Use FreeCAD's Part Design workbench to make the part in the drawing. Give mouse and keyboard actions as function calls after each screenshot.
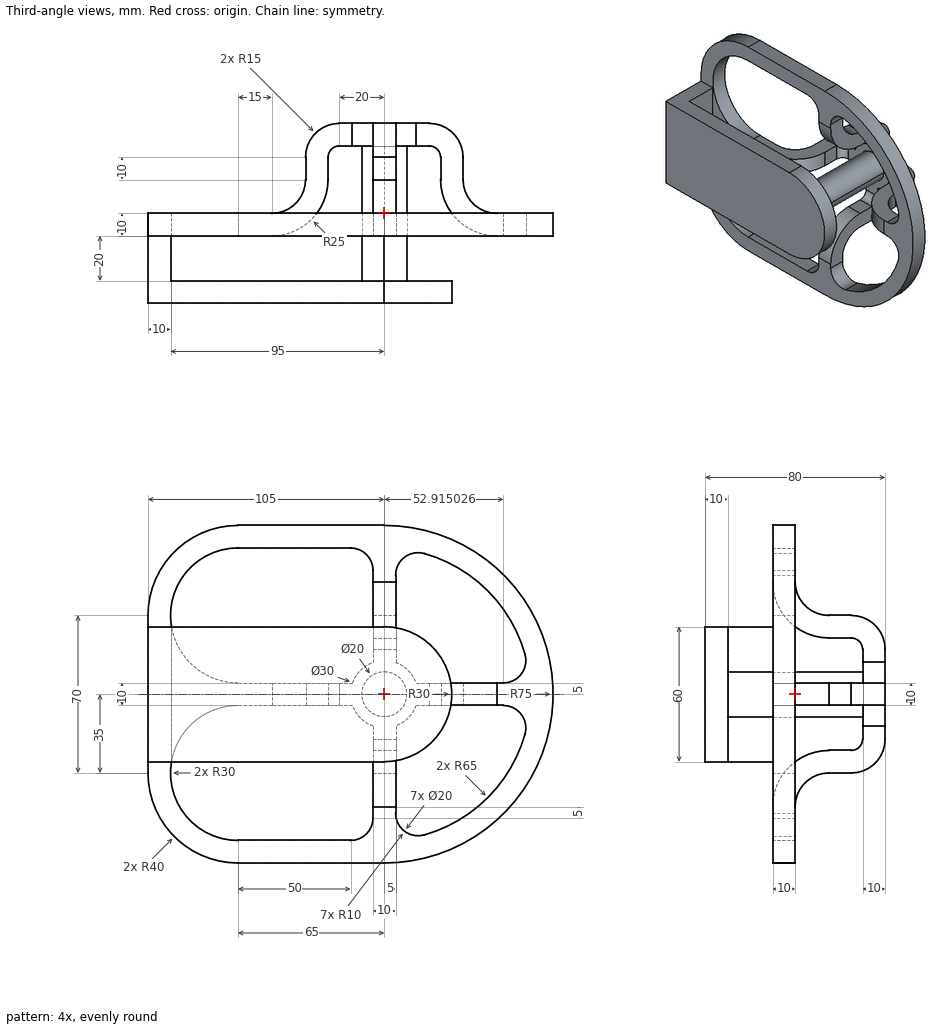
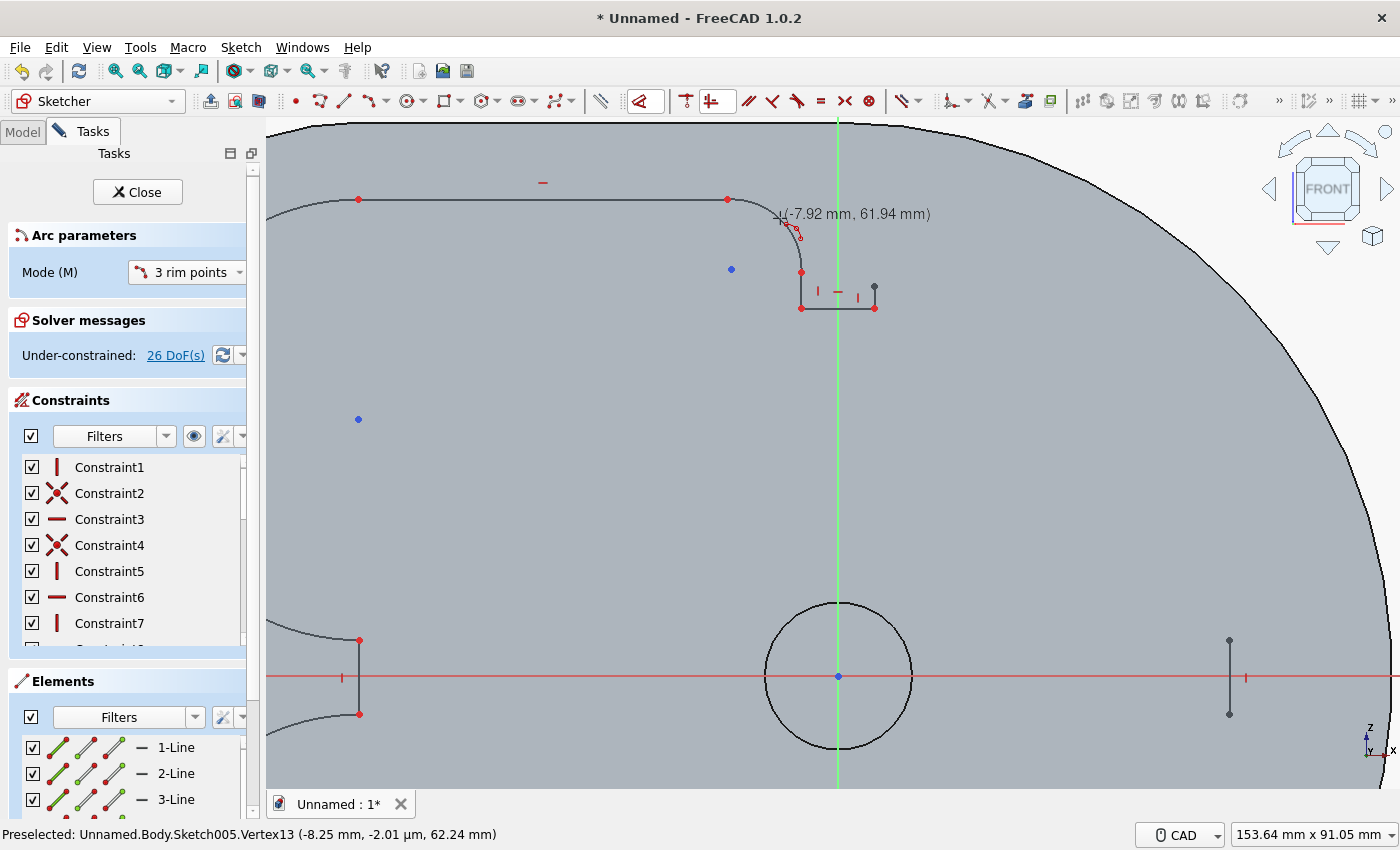
scroll(875, 286, up, 2)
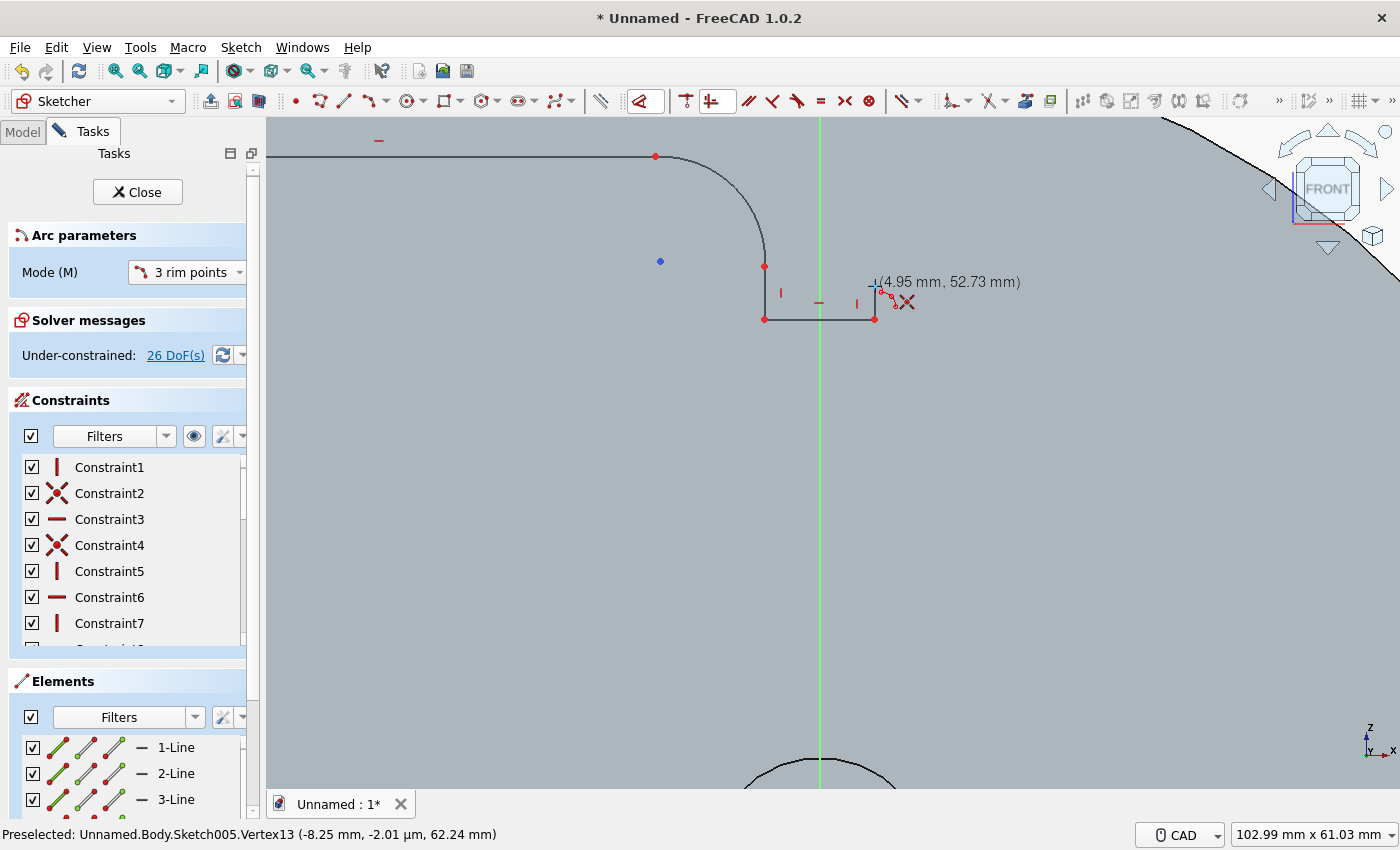
click(875, 287)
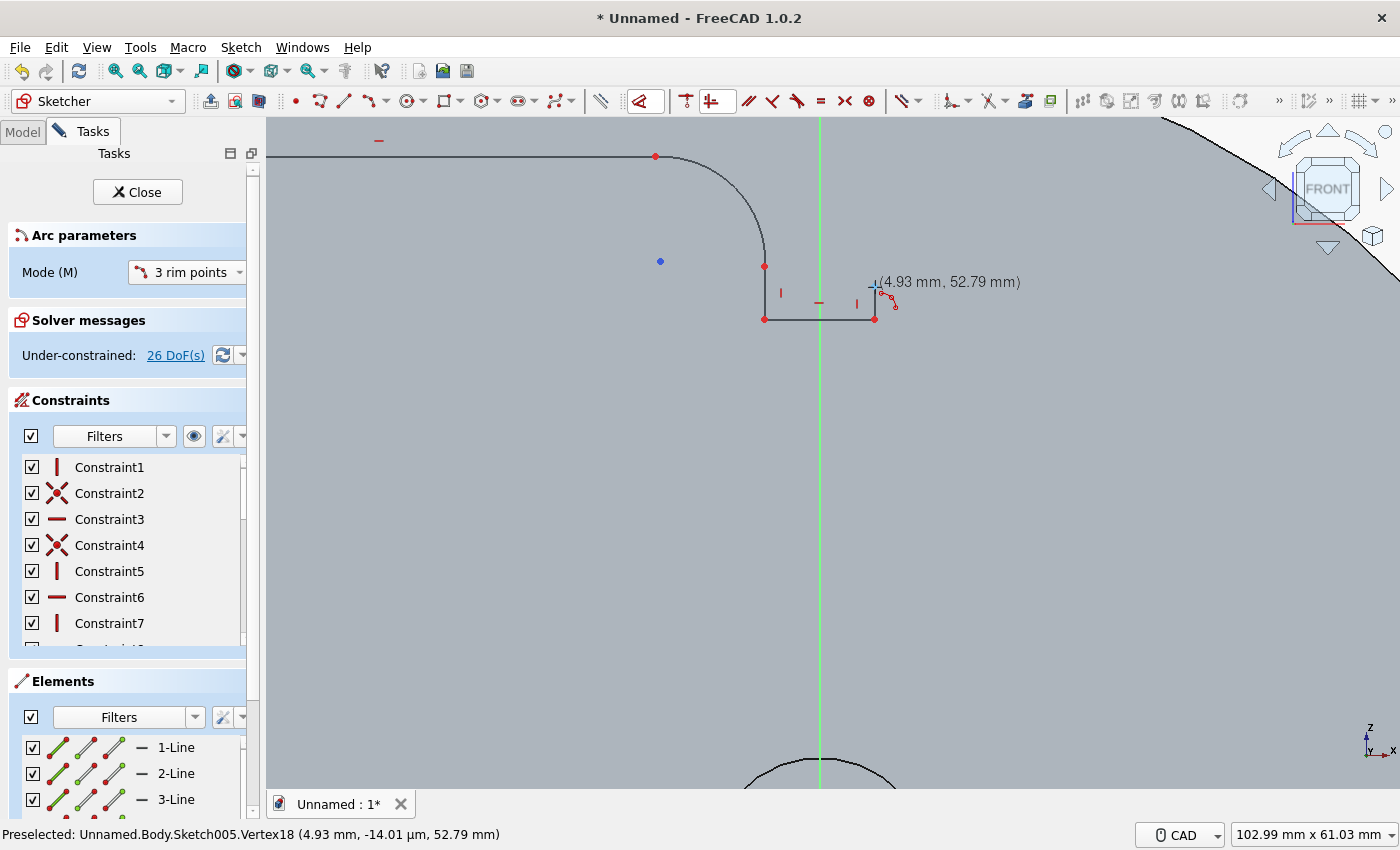
scroll(818, 274, down, 6)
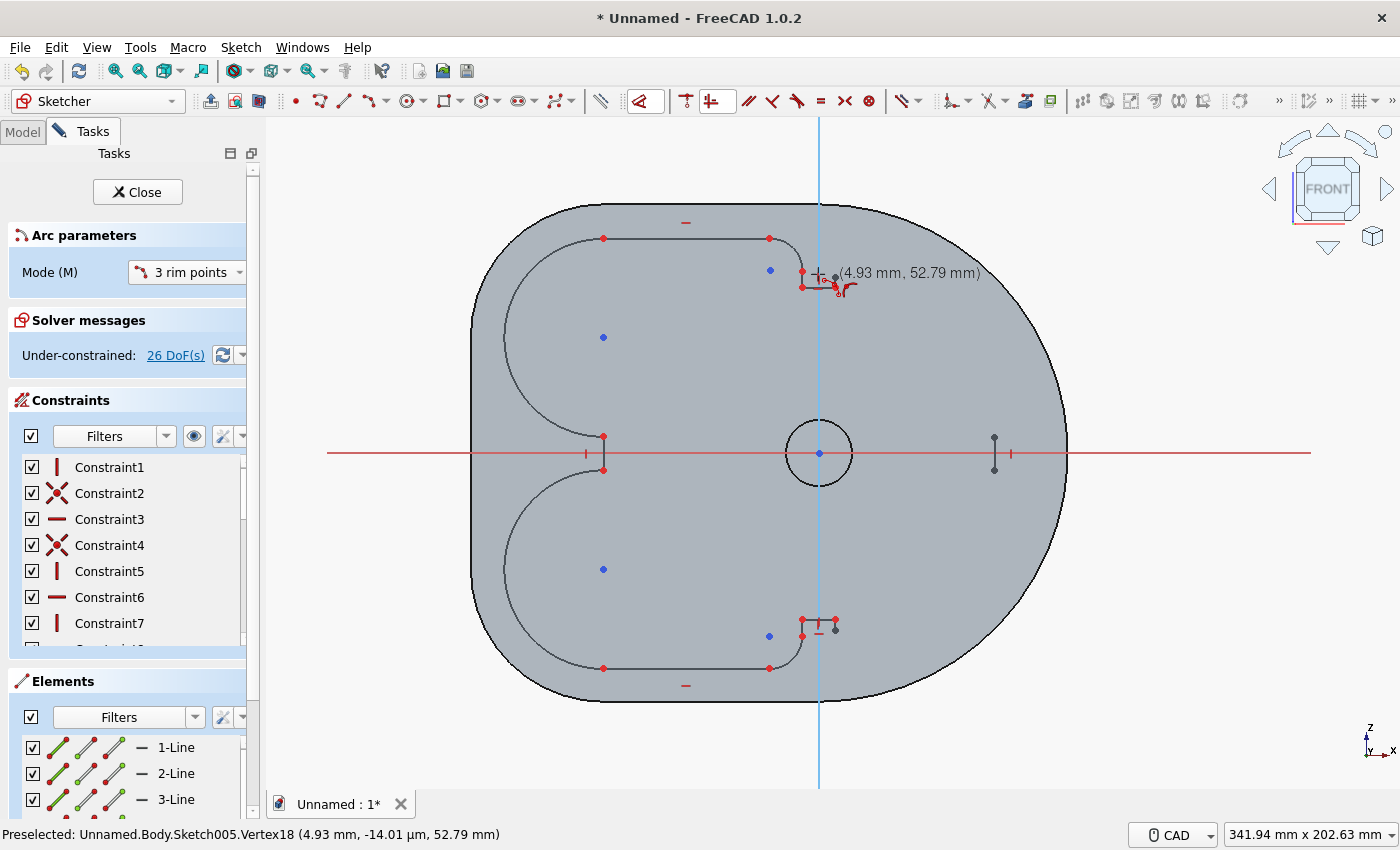
click(878, 246)
click(849, 251)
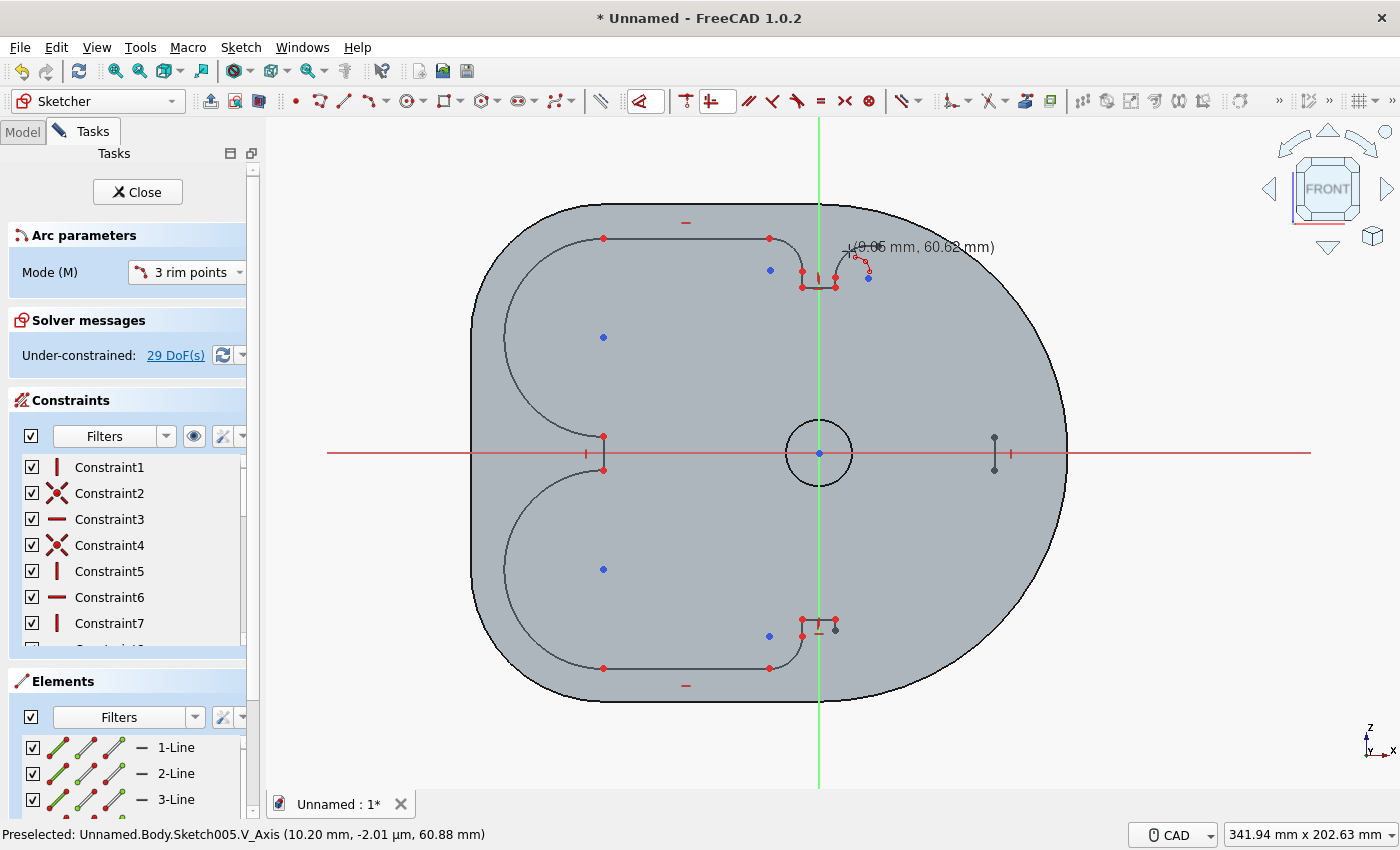
click(878, 247)
click(1026, 394)
click(971, 301)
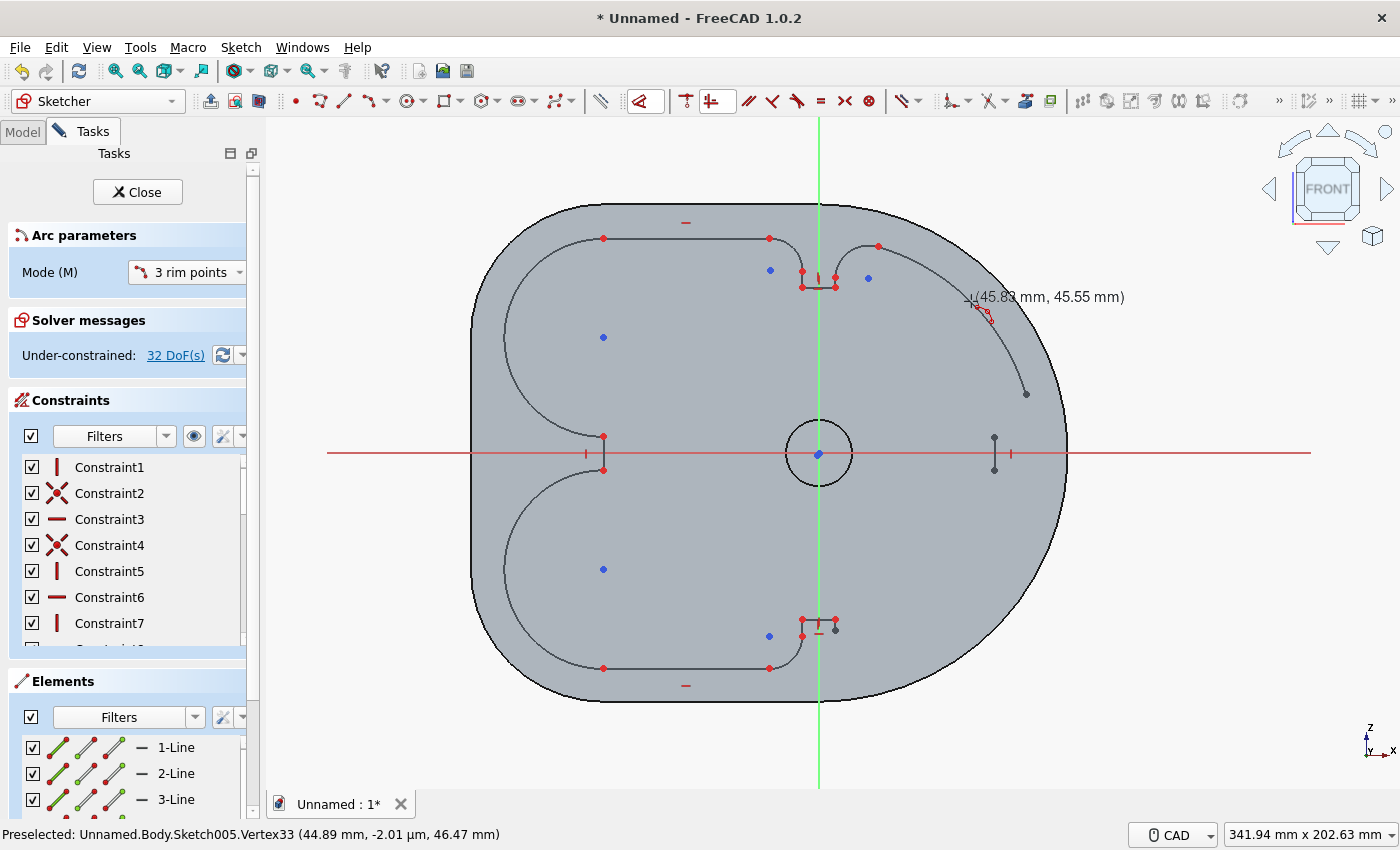
click(1026, 395)
click(995, 437)
click(1021, 423)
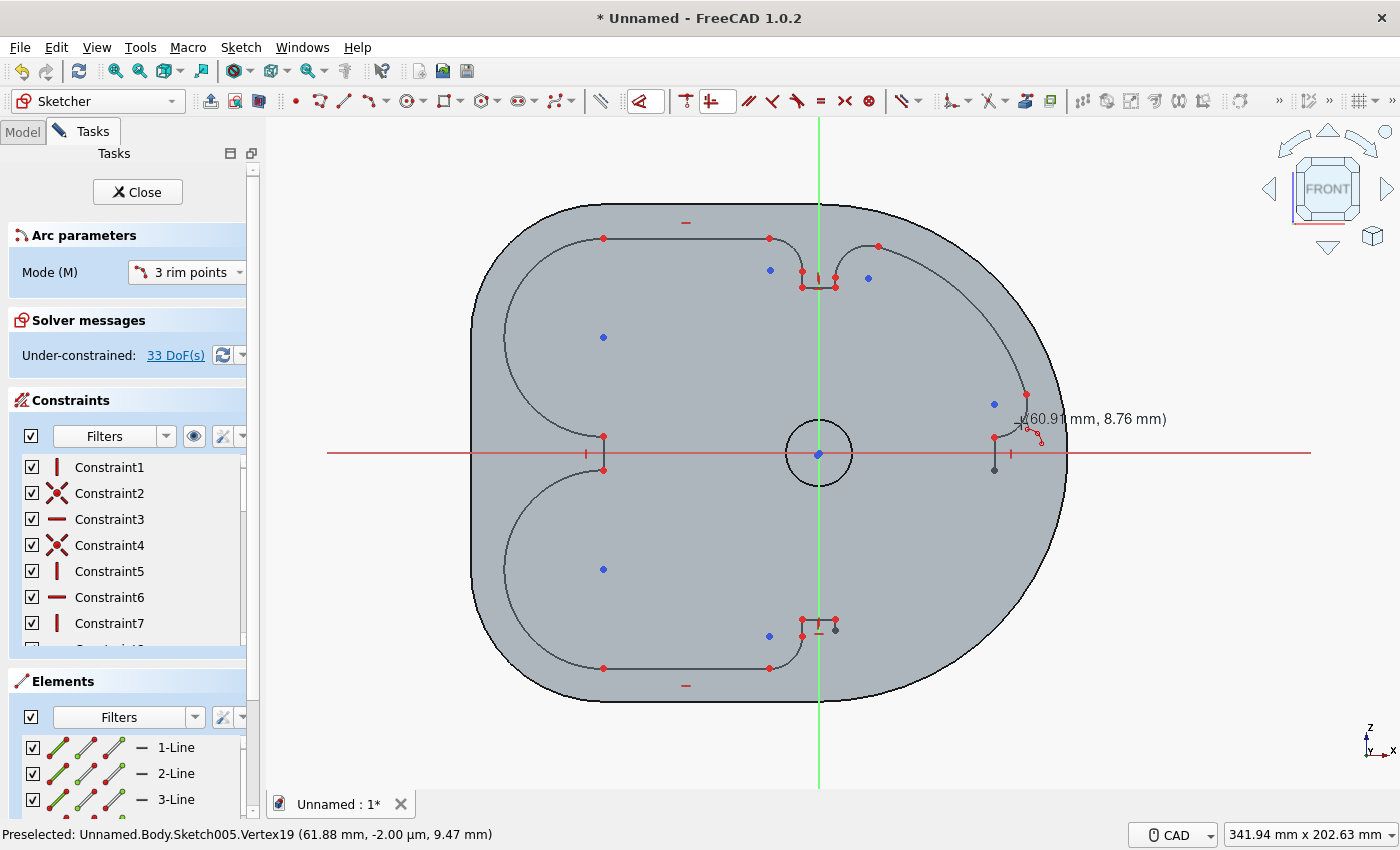
click(995, 470)
click(1026, 512)
click(1021, 483)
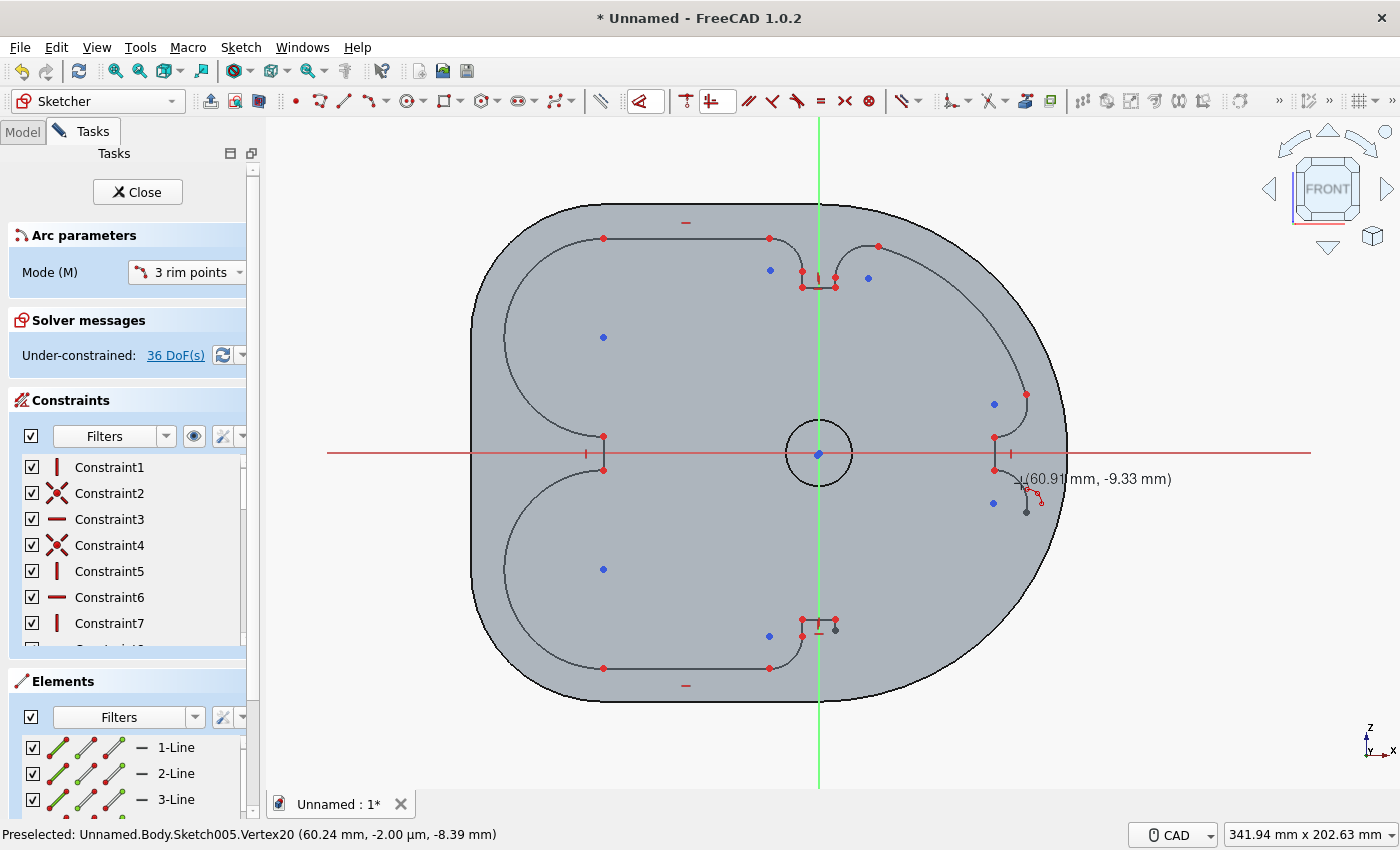
click(1026, 513)
click(878, 660)
click(971, 605)